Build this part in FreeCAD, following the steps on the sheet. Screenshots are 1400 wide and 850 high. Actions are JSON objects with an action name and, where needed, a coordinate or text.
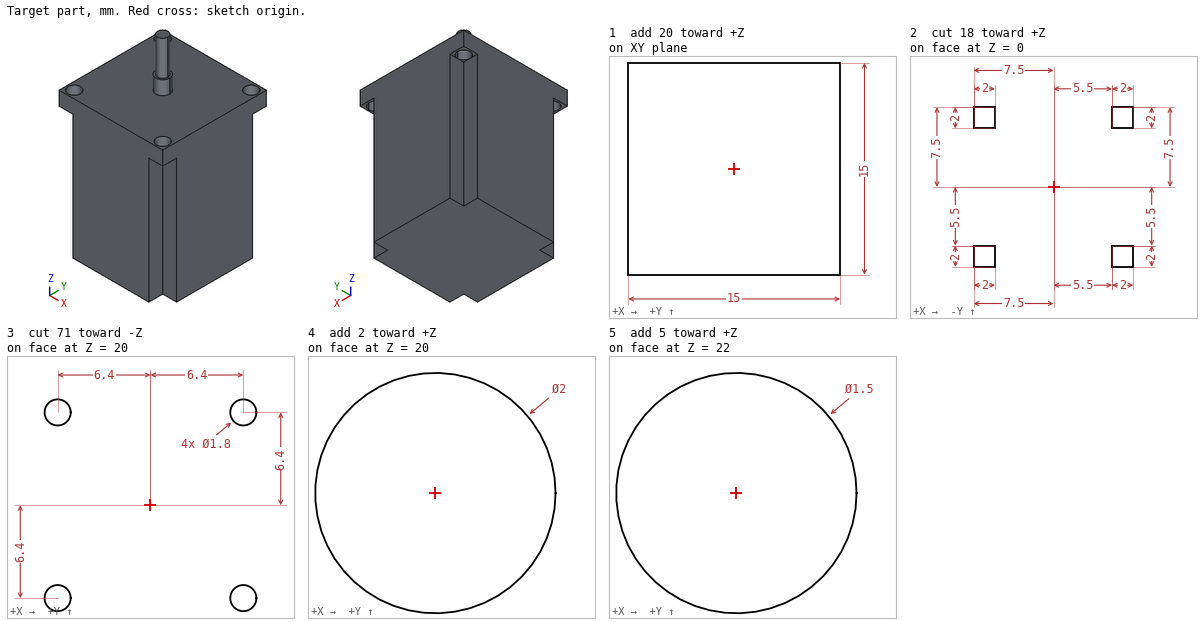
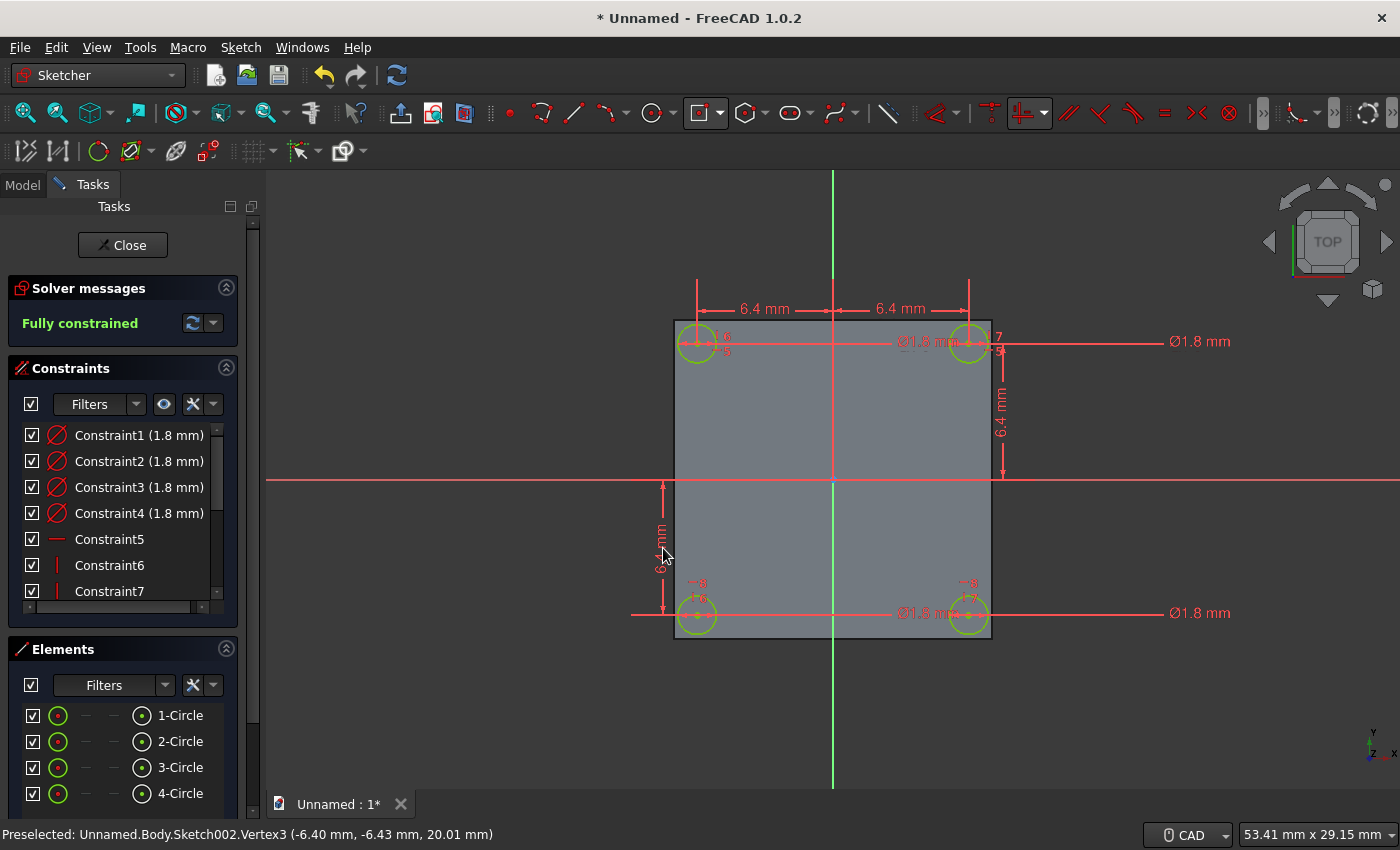
{"action": "left_click", "coordinate": [123, 245]}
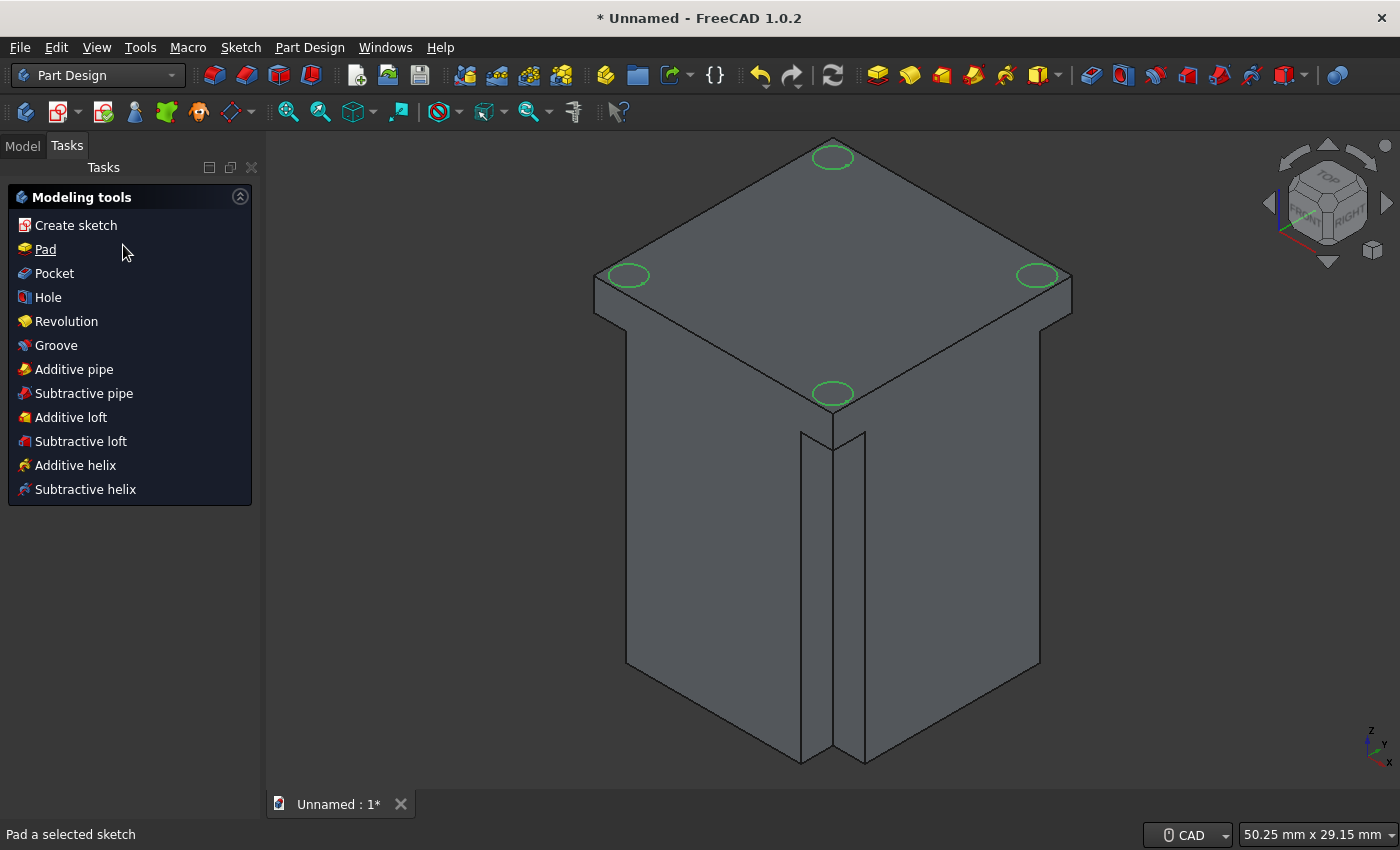
{"action": "left_click", "coordinate": [1092, 76]}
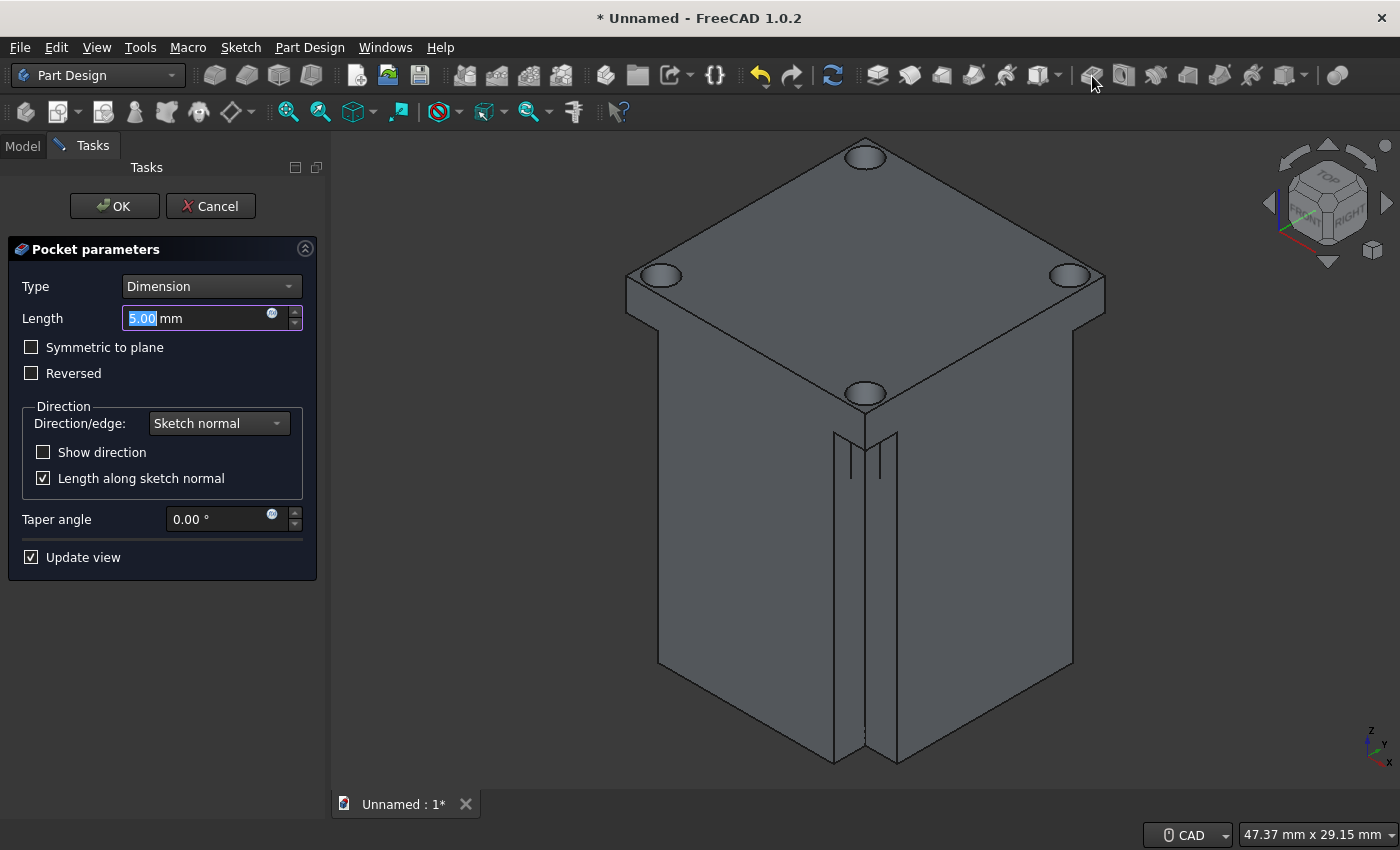
{"action": "type", "text": "71"}
{"action": "key", "text": "Tab"}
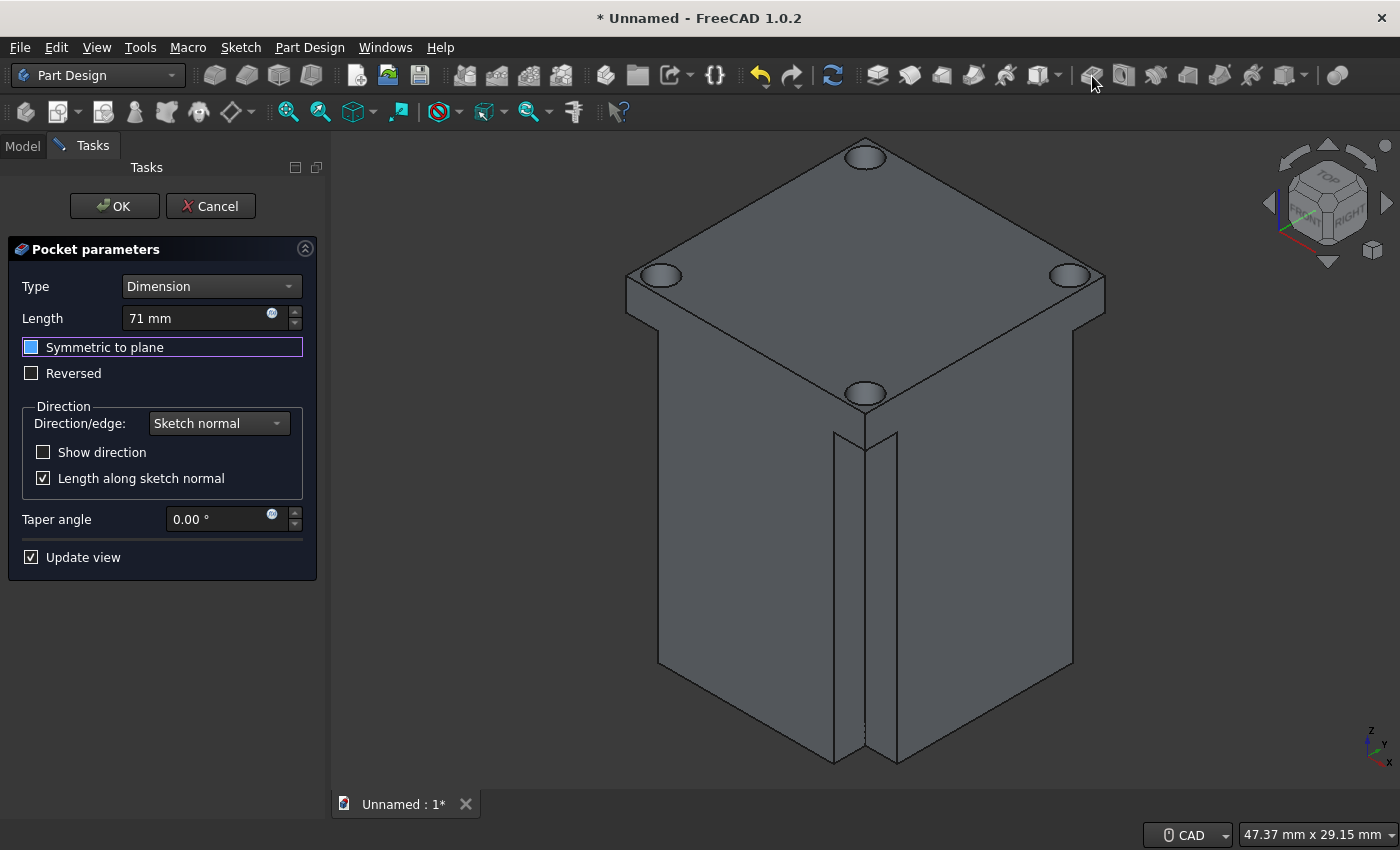
{"action": "left_click", "coordinate": [115, 206]}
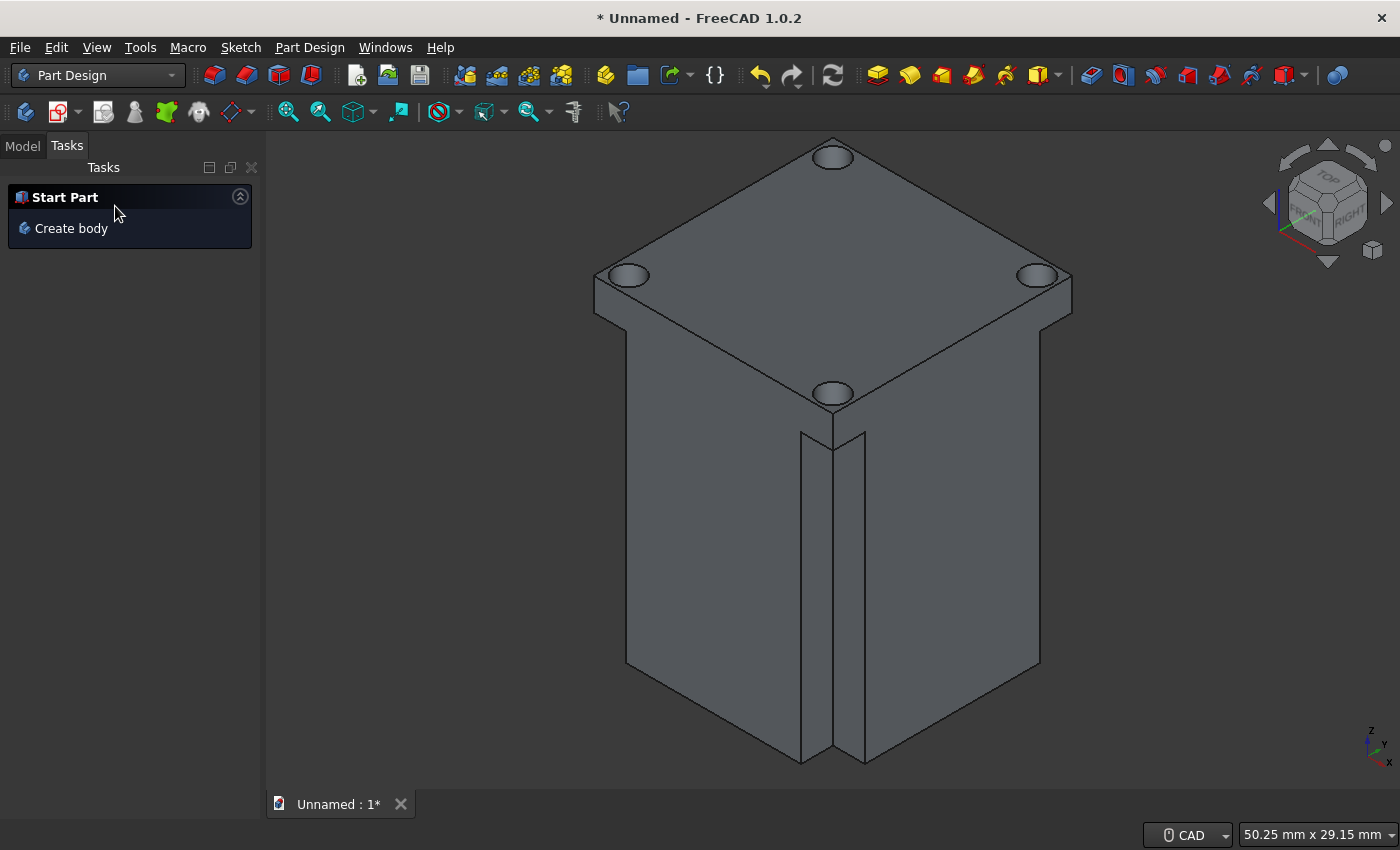
{"action": "left_click", "coordinate": [833, 275]}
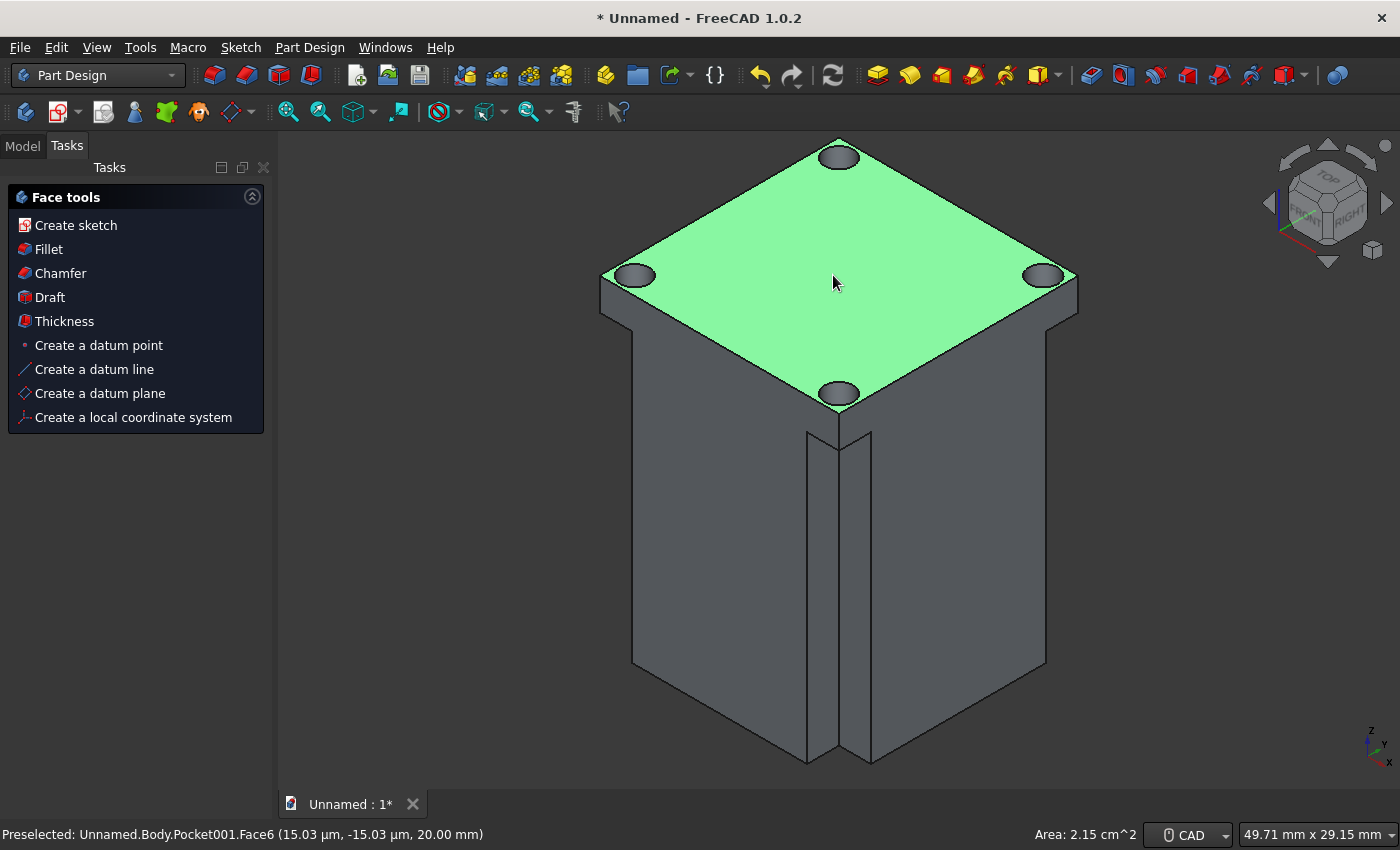
{"action": "left_click", "coordinate": [58, 112]}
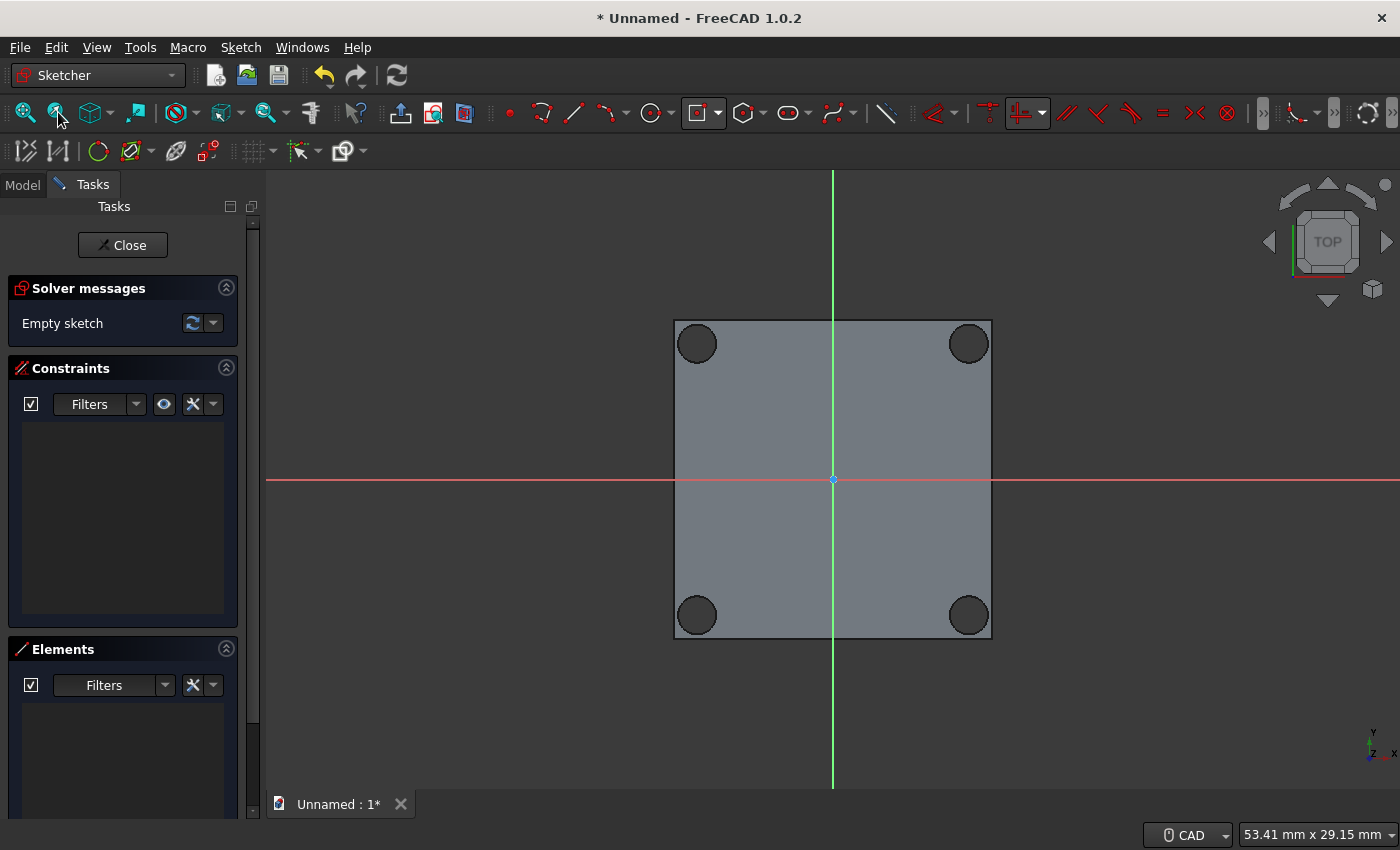
{"action": "scroll", "coordinate": [842, 479], "scroll_direction": "up", "scroll_amount": 11}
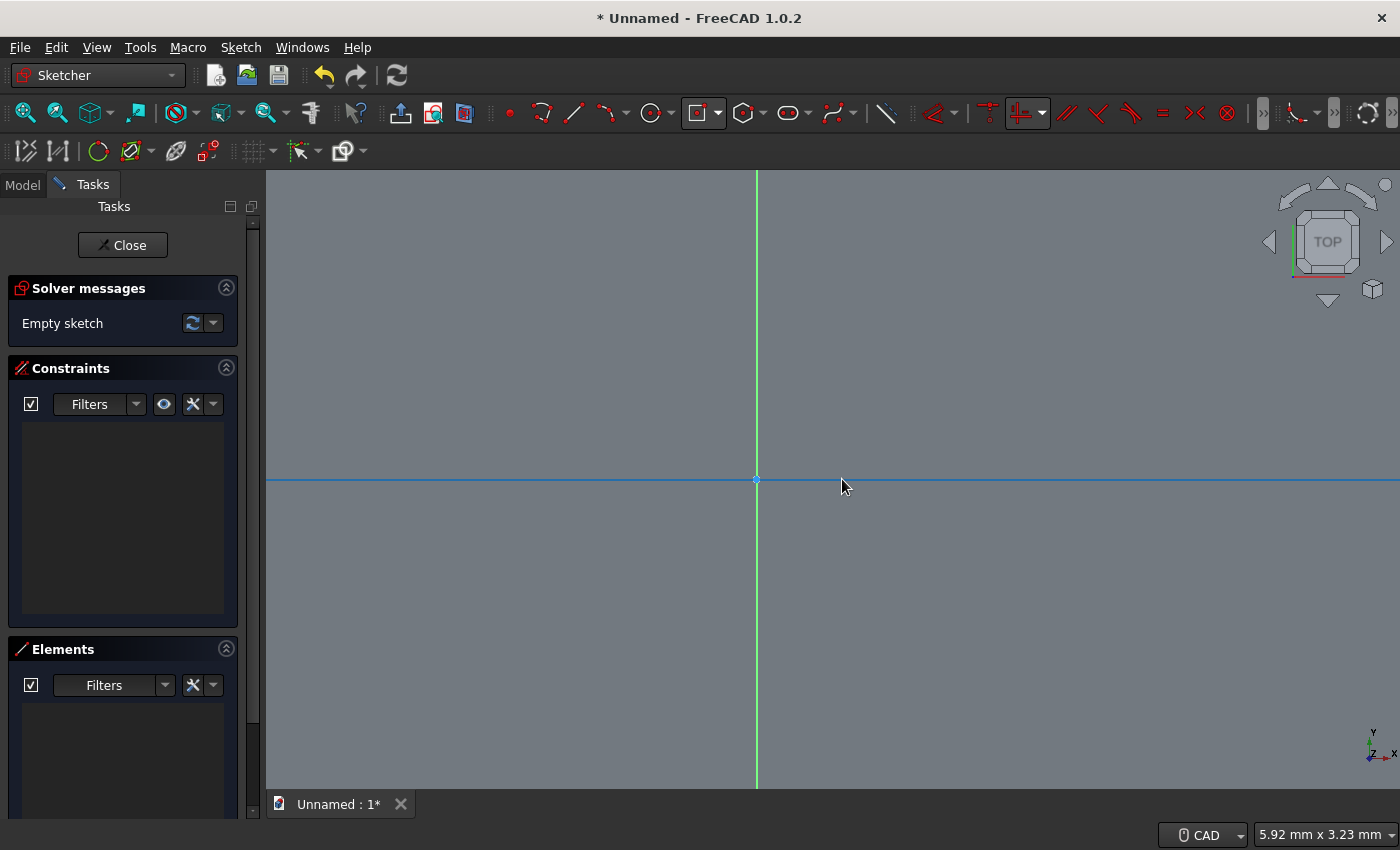
{"action": "left_click", "coordinate": [652, 114]}